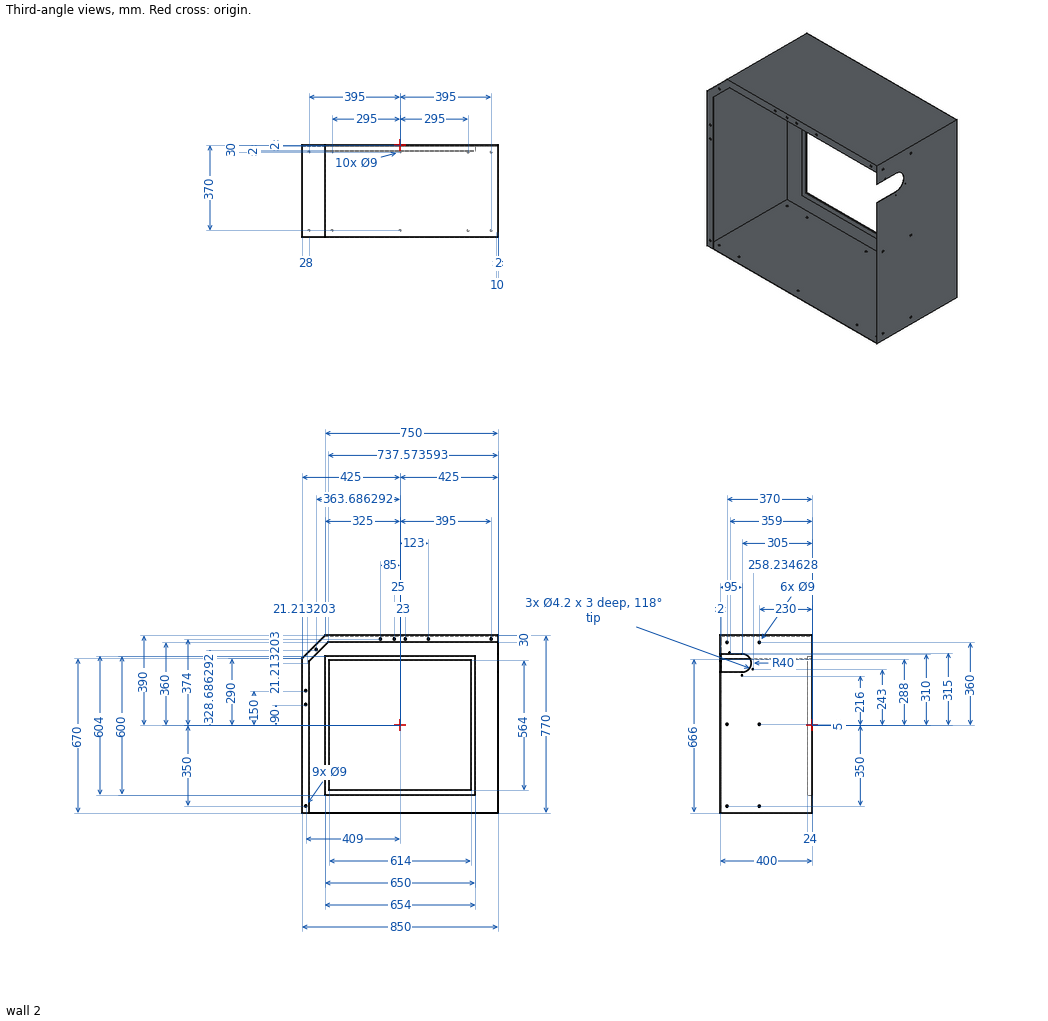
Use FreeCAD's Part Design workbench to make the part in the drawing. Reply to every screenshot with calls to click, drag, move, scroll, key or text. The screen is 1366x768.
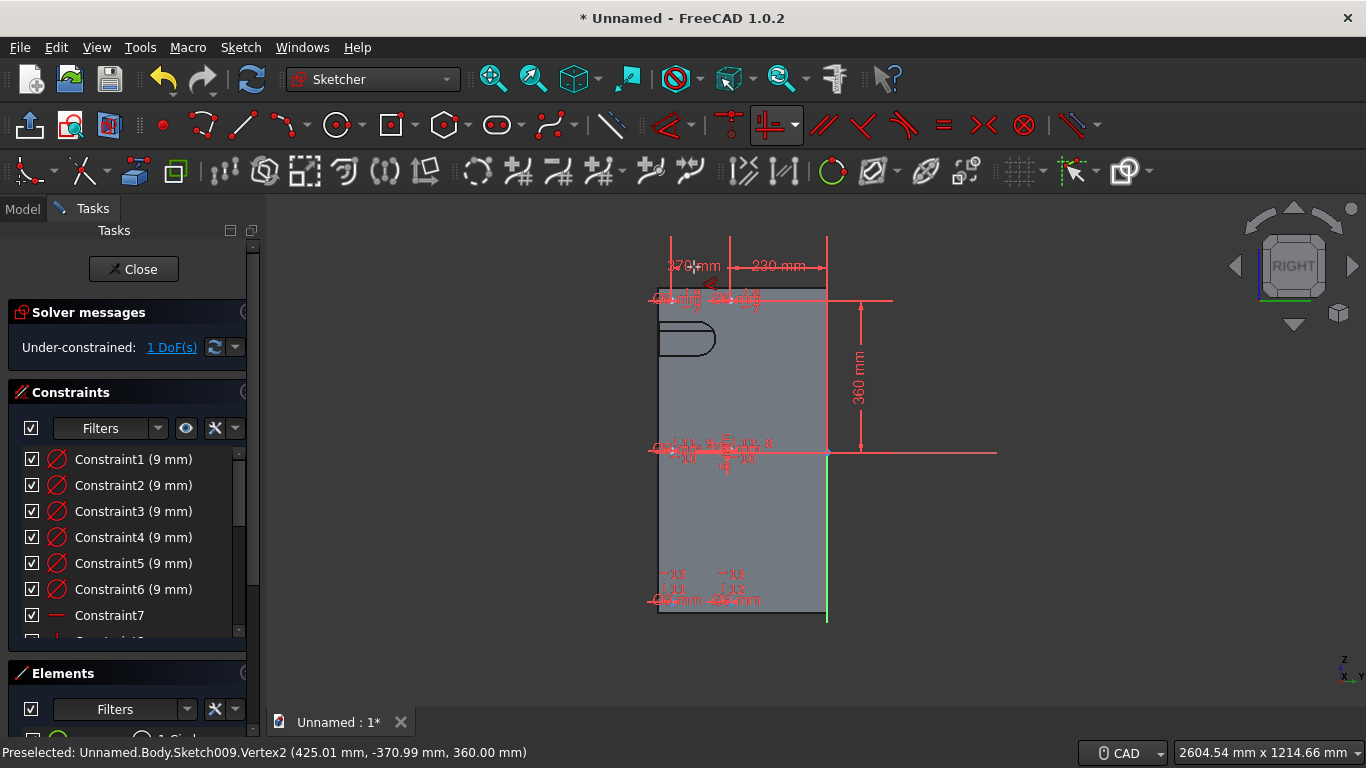
click(671, 602)
click(861, 527)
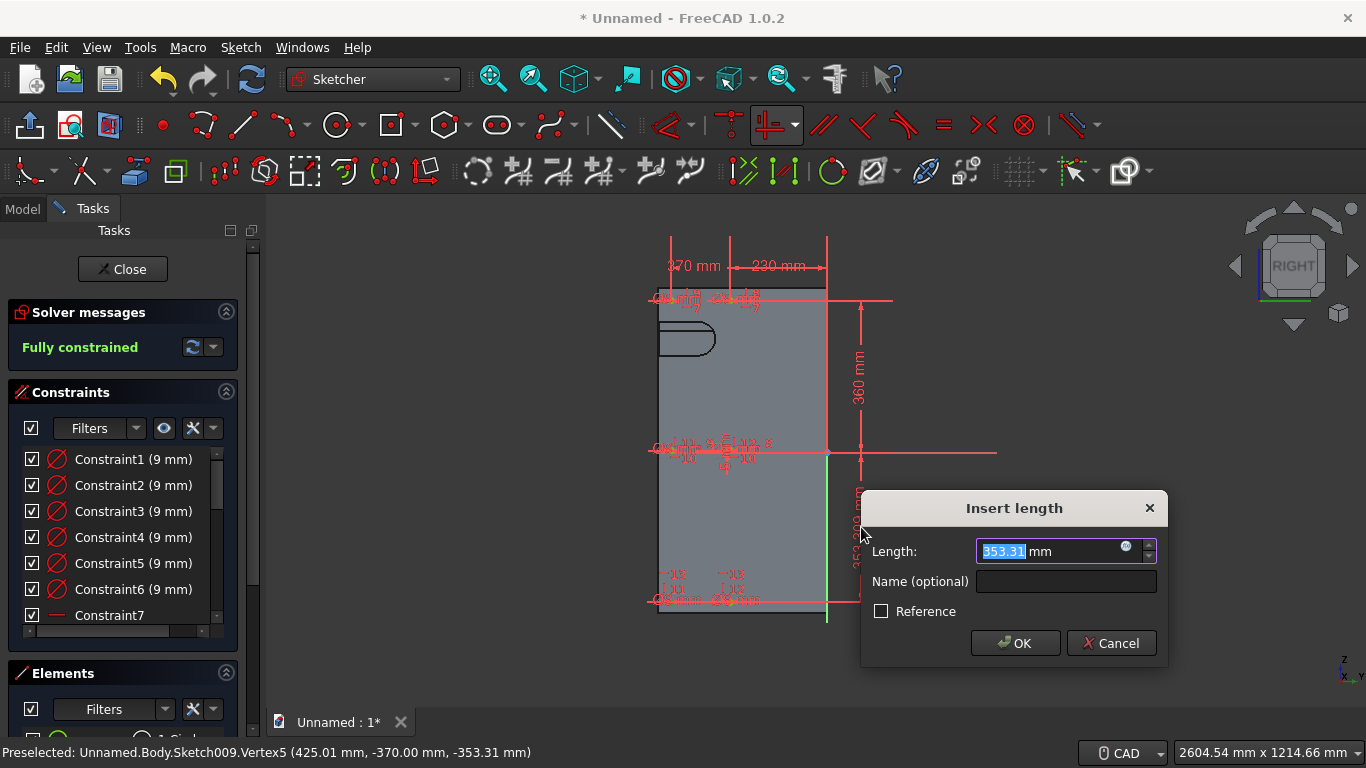
text(350)
key(Return)
key(Escape)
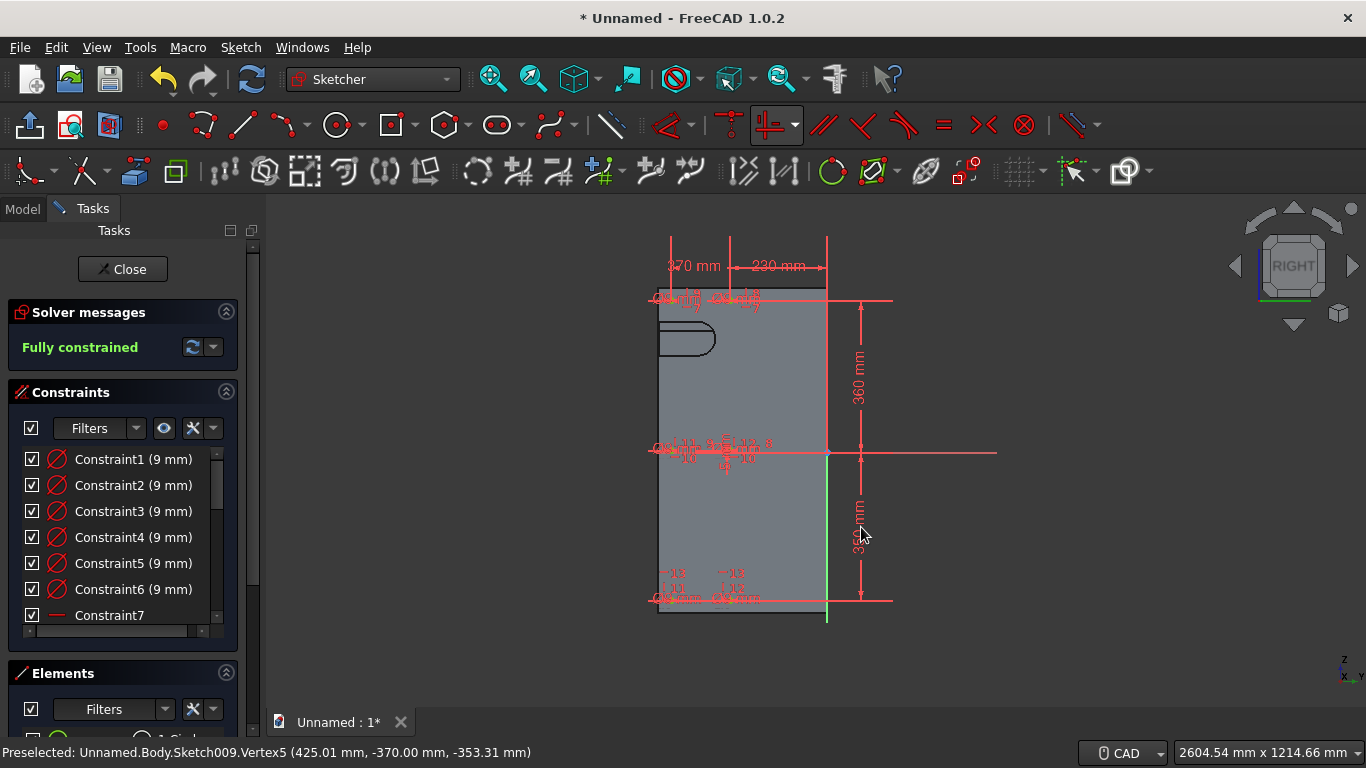
click(123, 269)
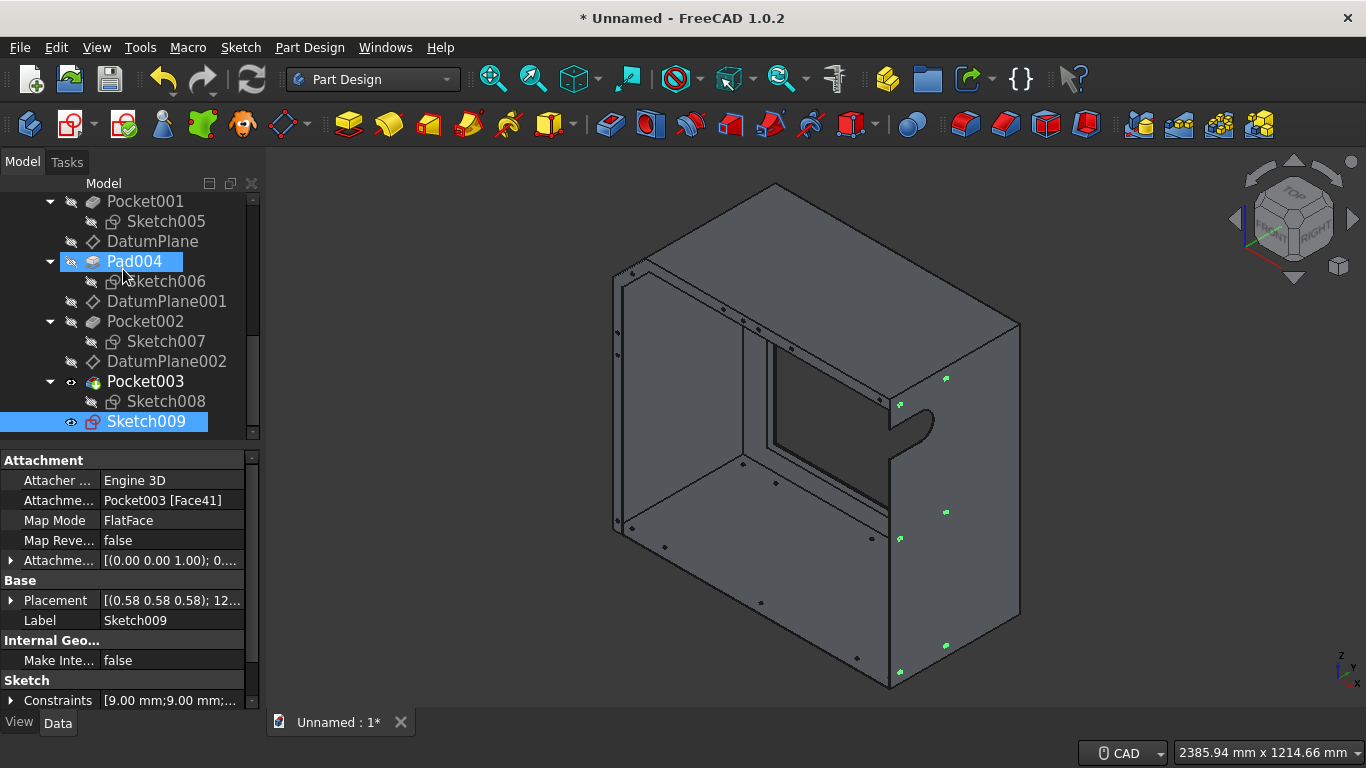
click(612, 124)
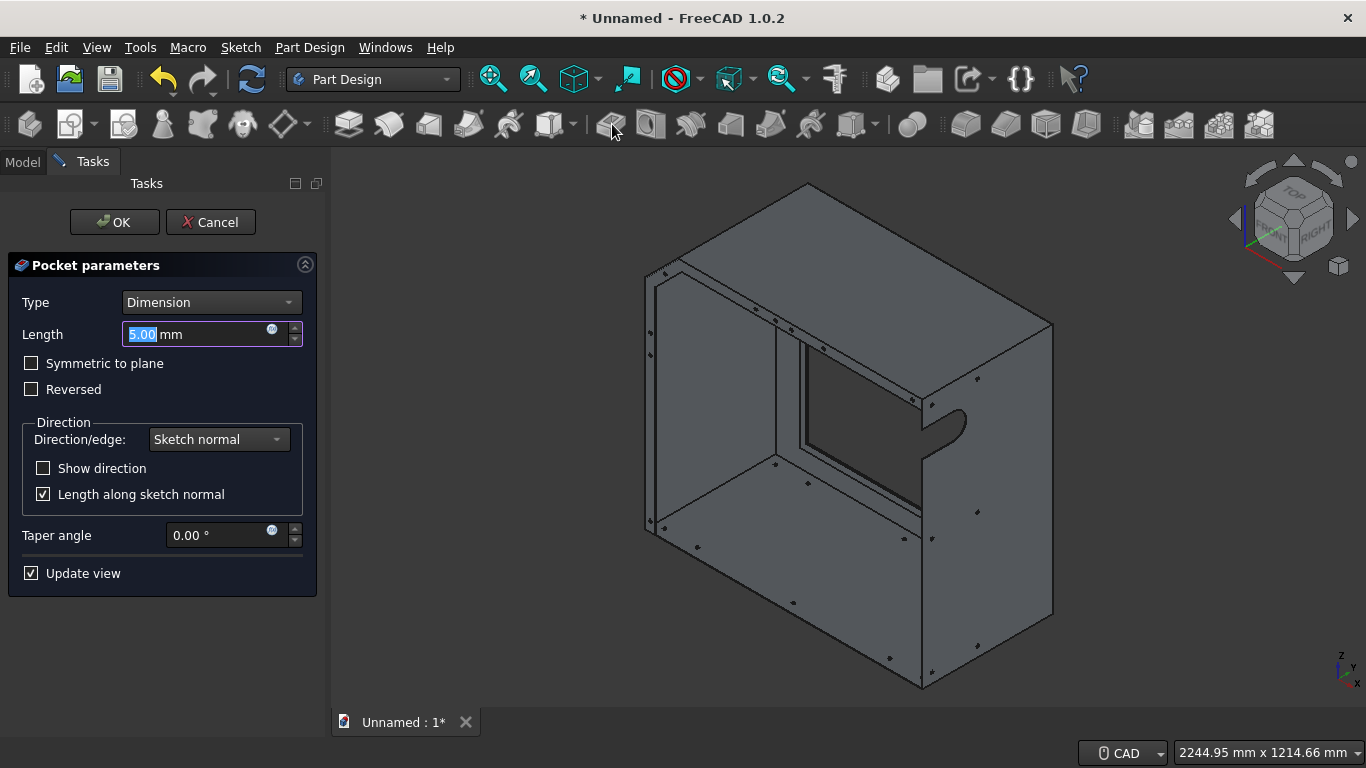
text(10)
key(Tab)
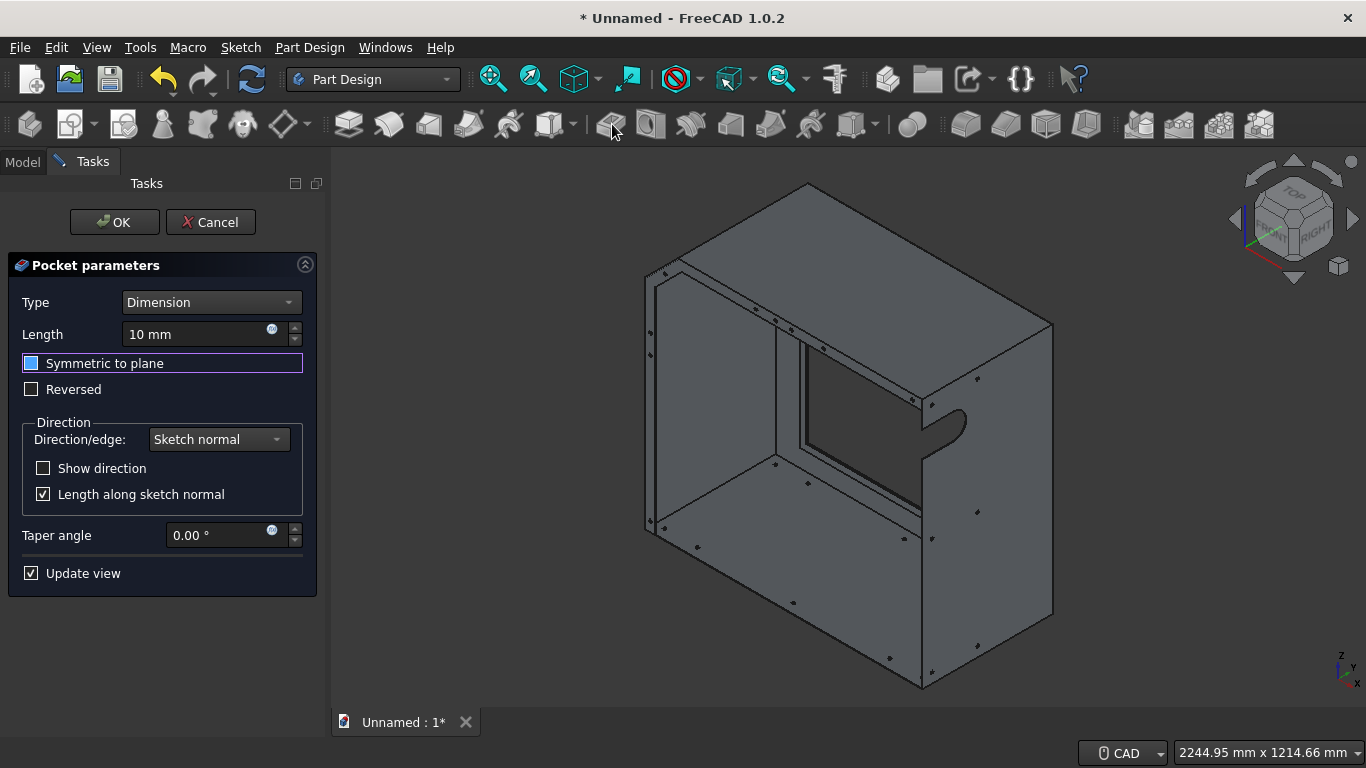
click(115, 222)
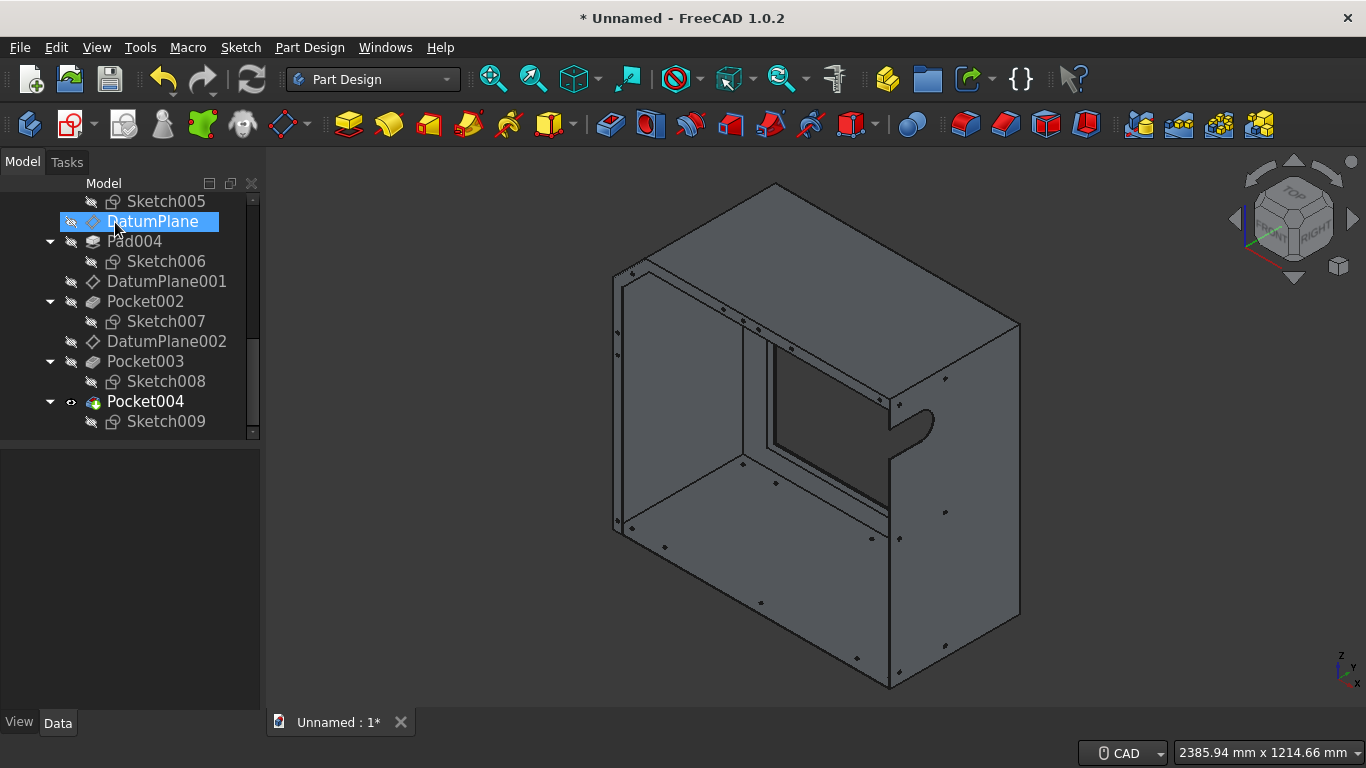
click(974, 578)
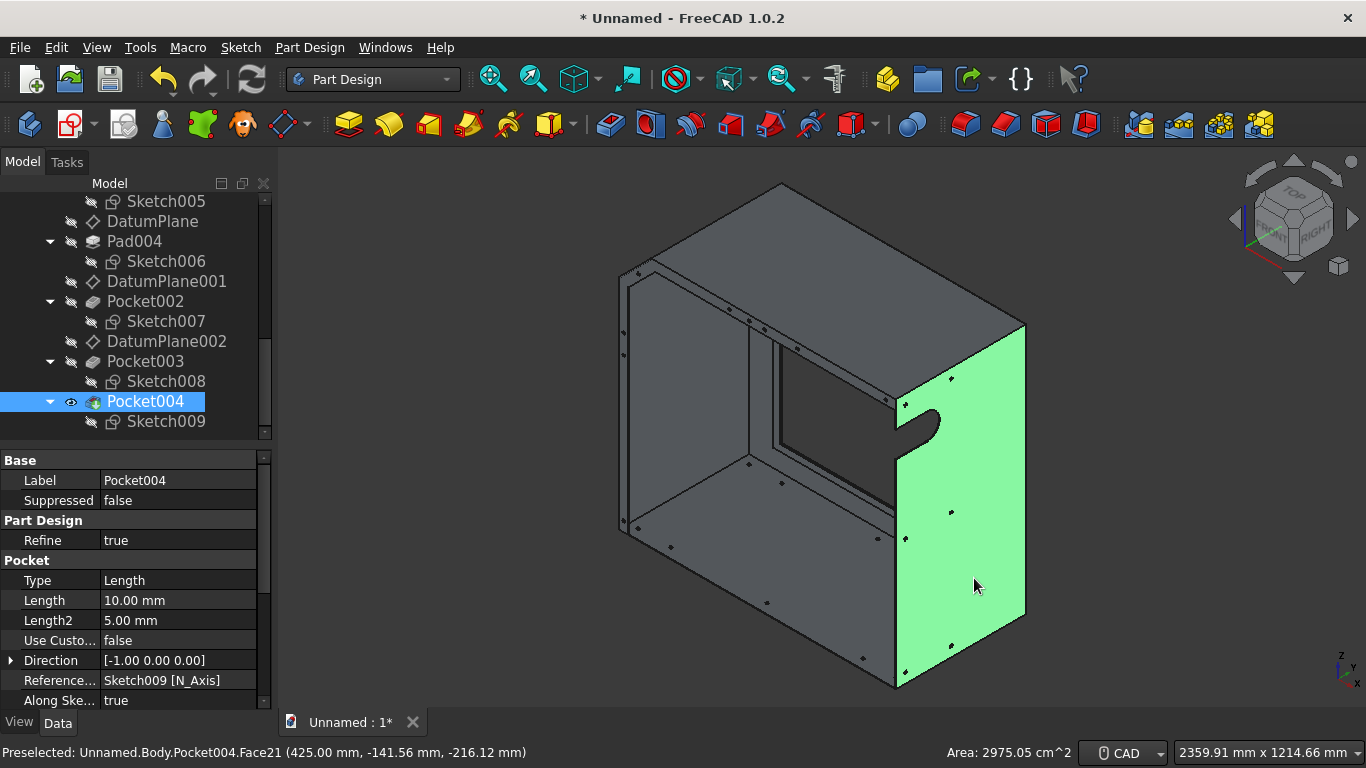
click(70, 124)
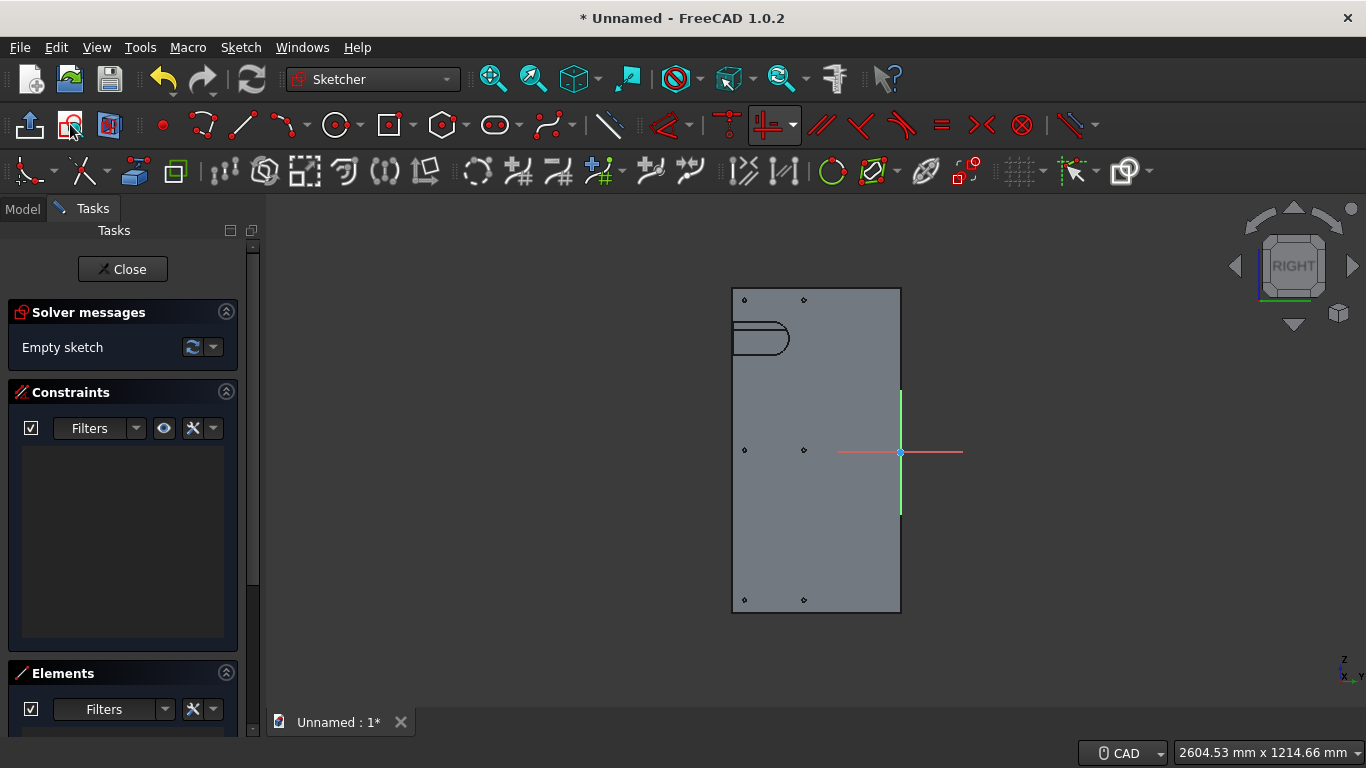
scroll(774, 323, up, 10)